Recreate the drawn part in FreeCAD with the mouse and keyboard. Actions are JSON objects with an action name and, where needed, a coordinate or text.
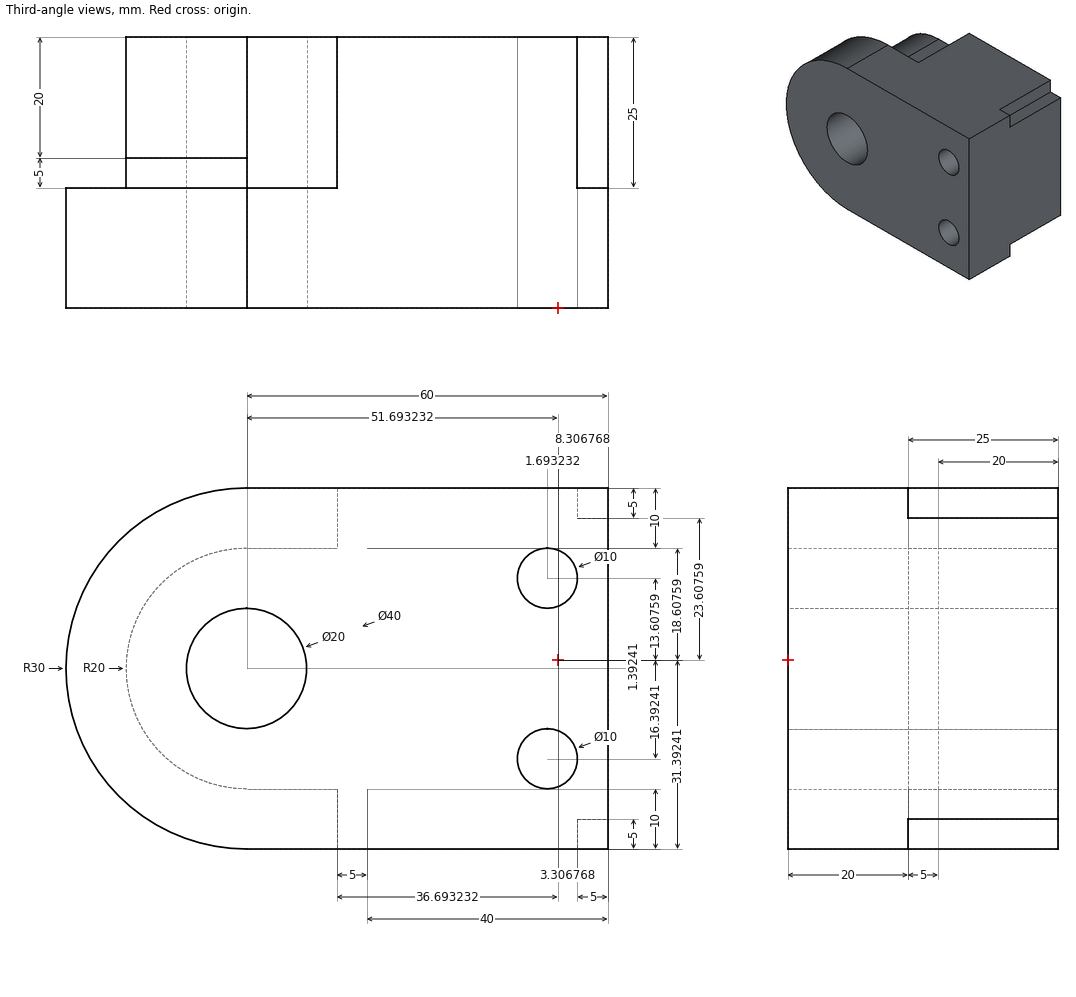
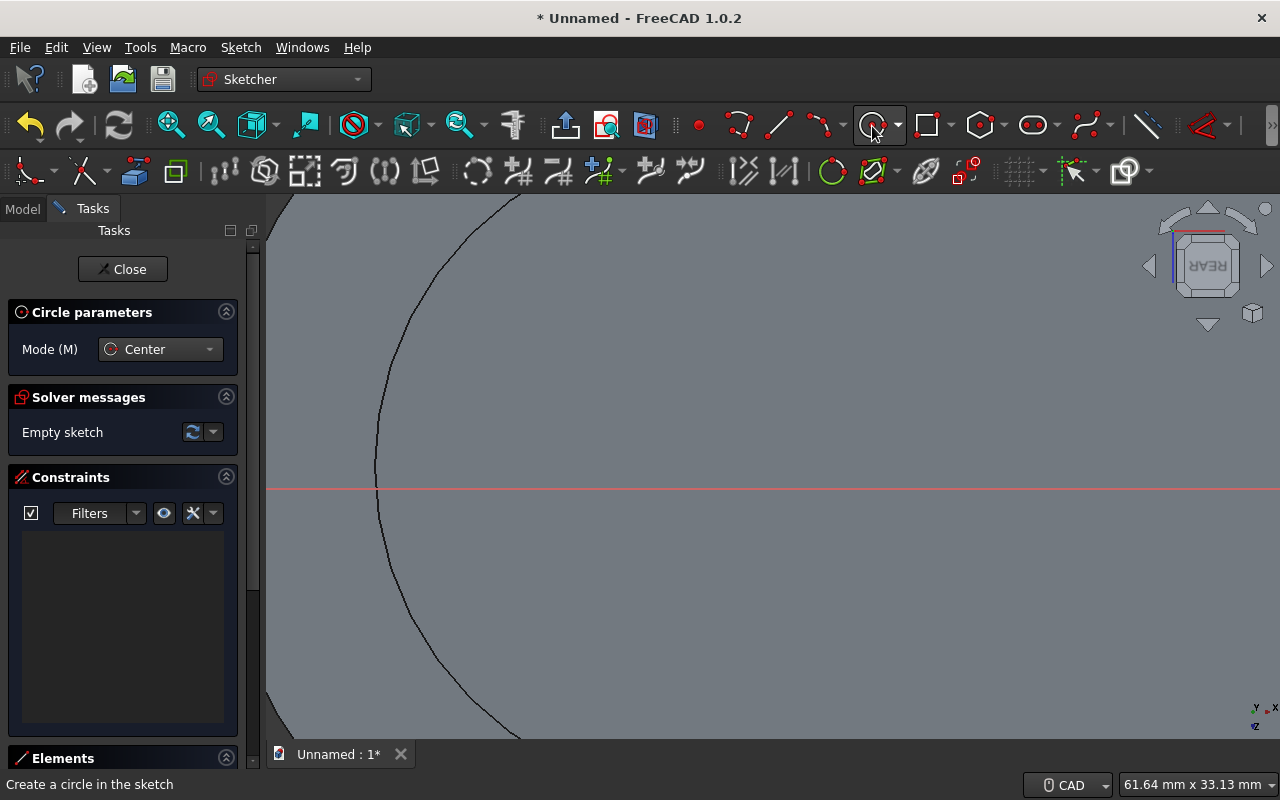
{"action": "left_click", "coordinate": [704, 466]}
{"action": "left_click", "coordinate": [820, 350]}
{"action": "key", "text": "Escape"}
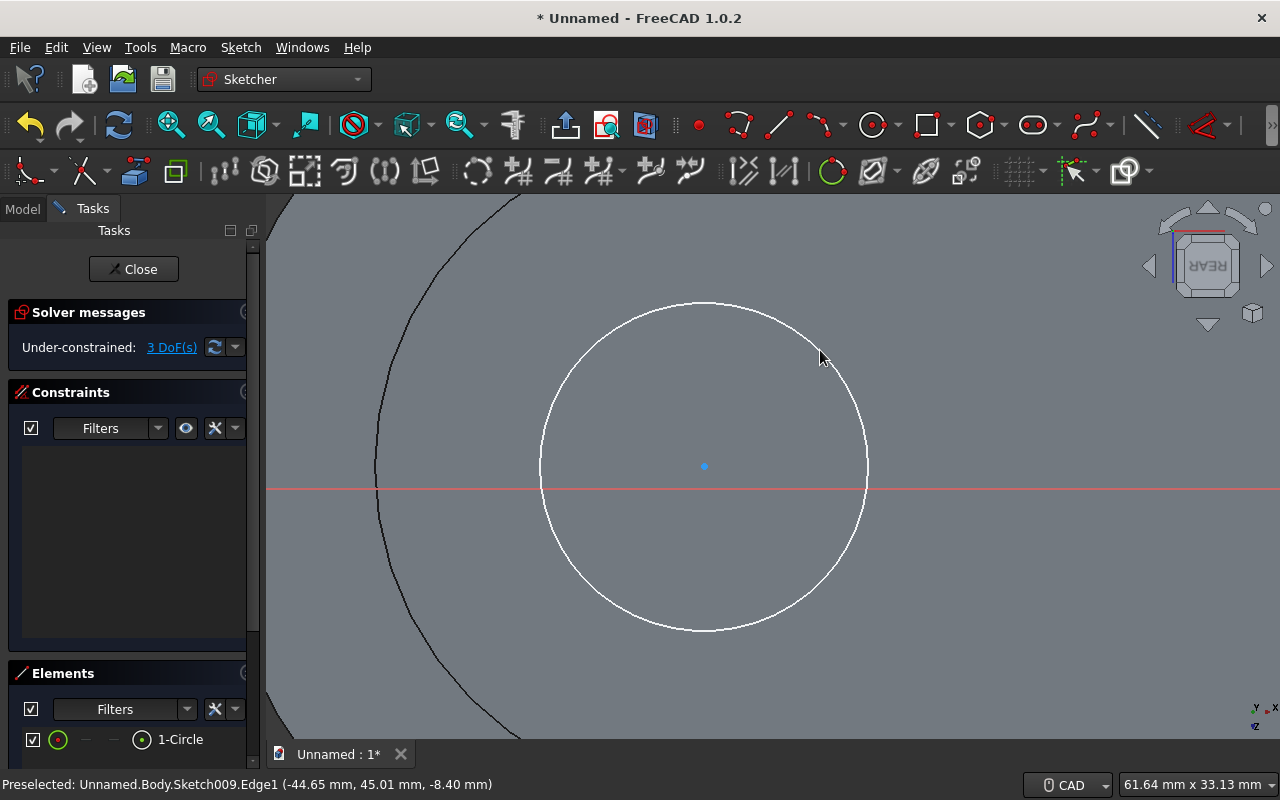
{"action": "left_click", "coordinate": [1202, 126]}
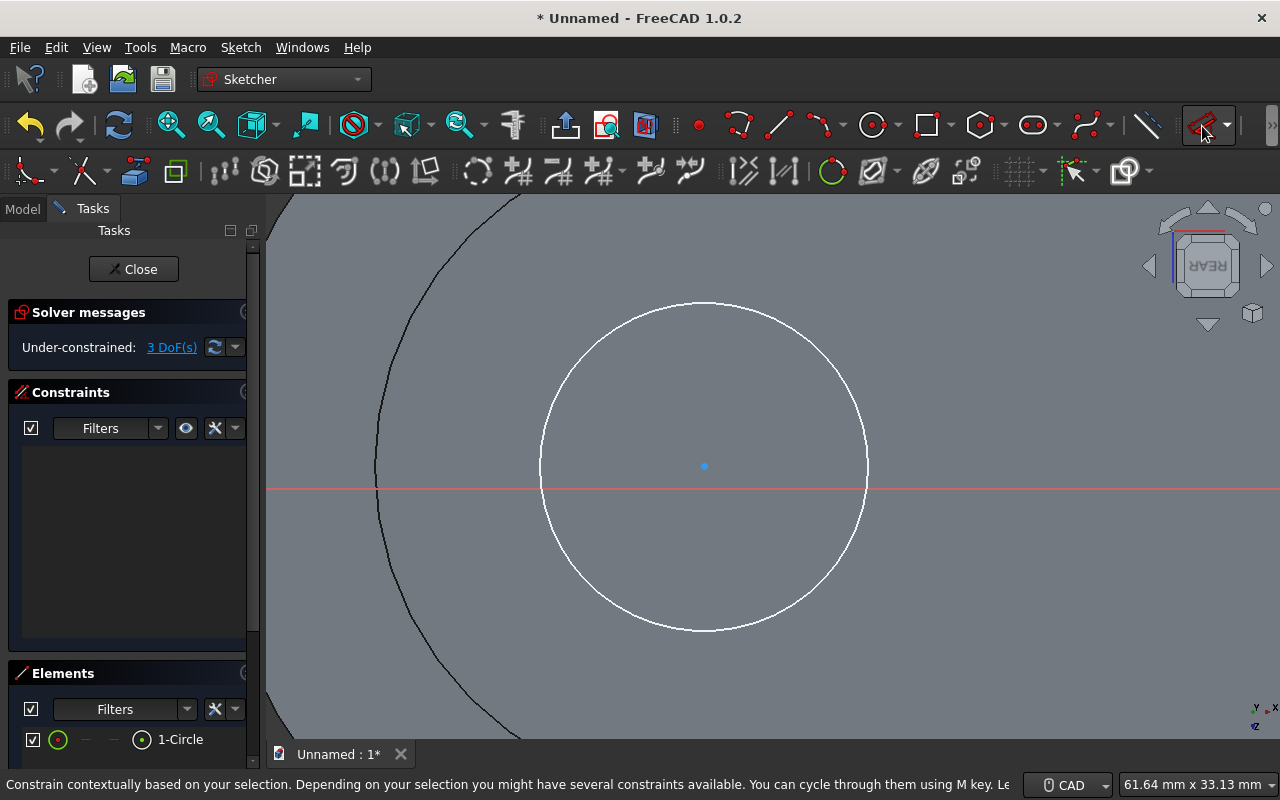
{"action": "left_click", "coordinate": [820, 351]}
{"action": "left_click", "coordinate": [843, 328]}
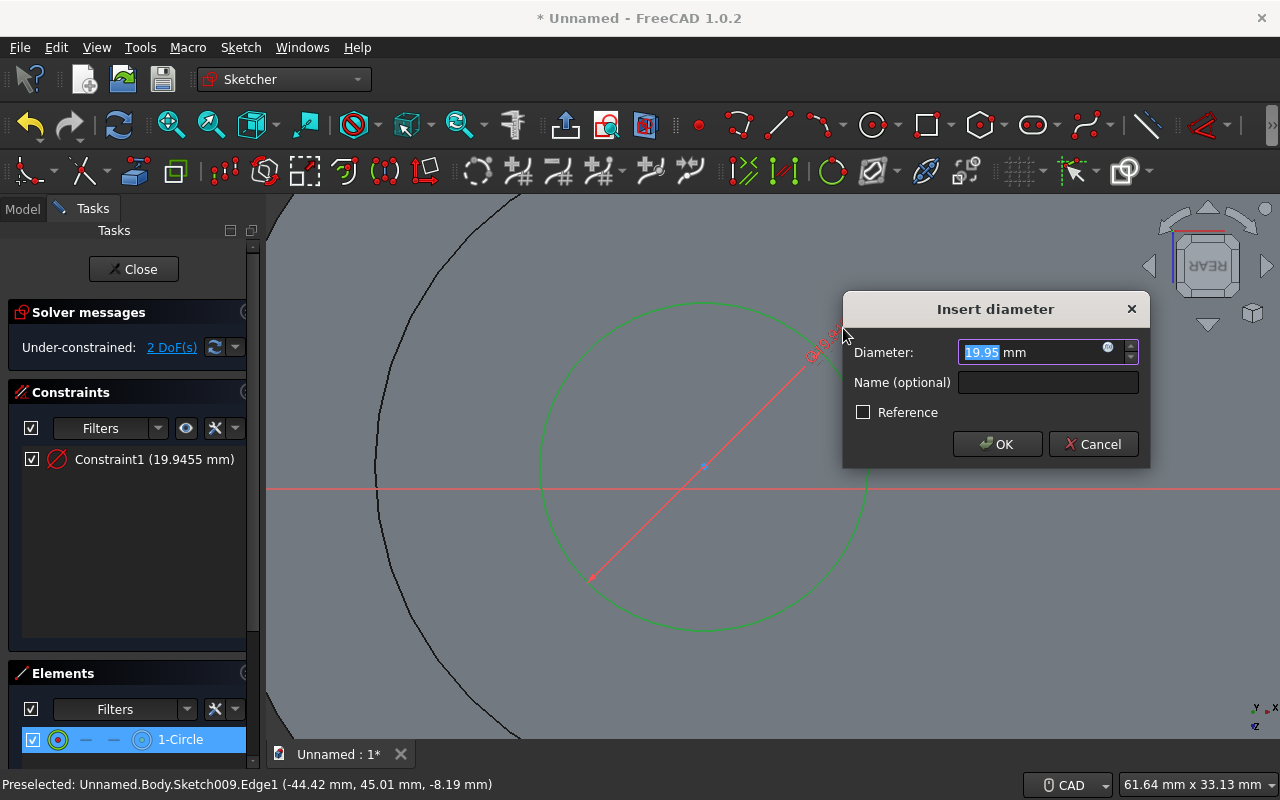
{"action": "type", "text": "20"}
{"action": "key", "text": "Return"}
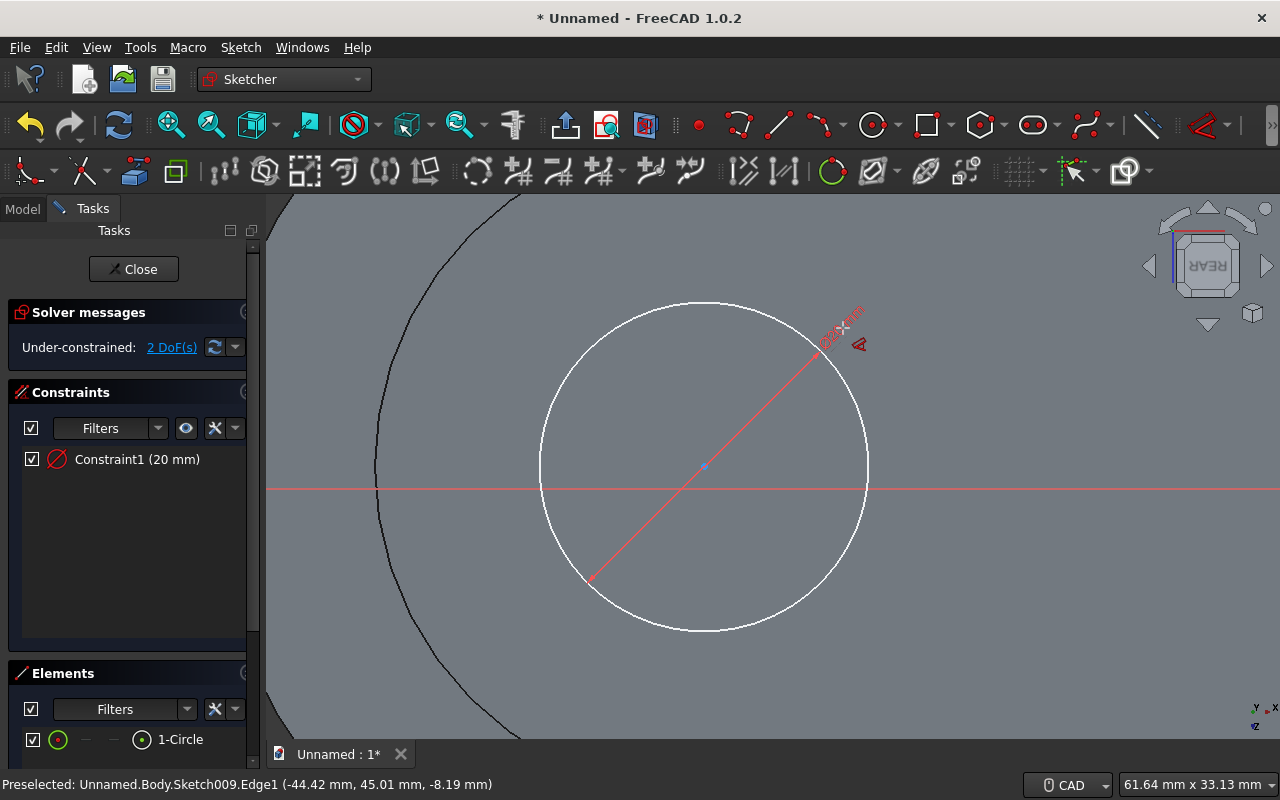
{"action": "scroll", "coordinate": [704, 467], "scroll_direction": "up", "scroll_amount": 3}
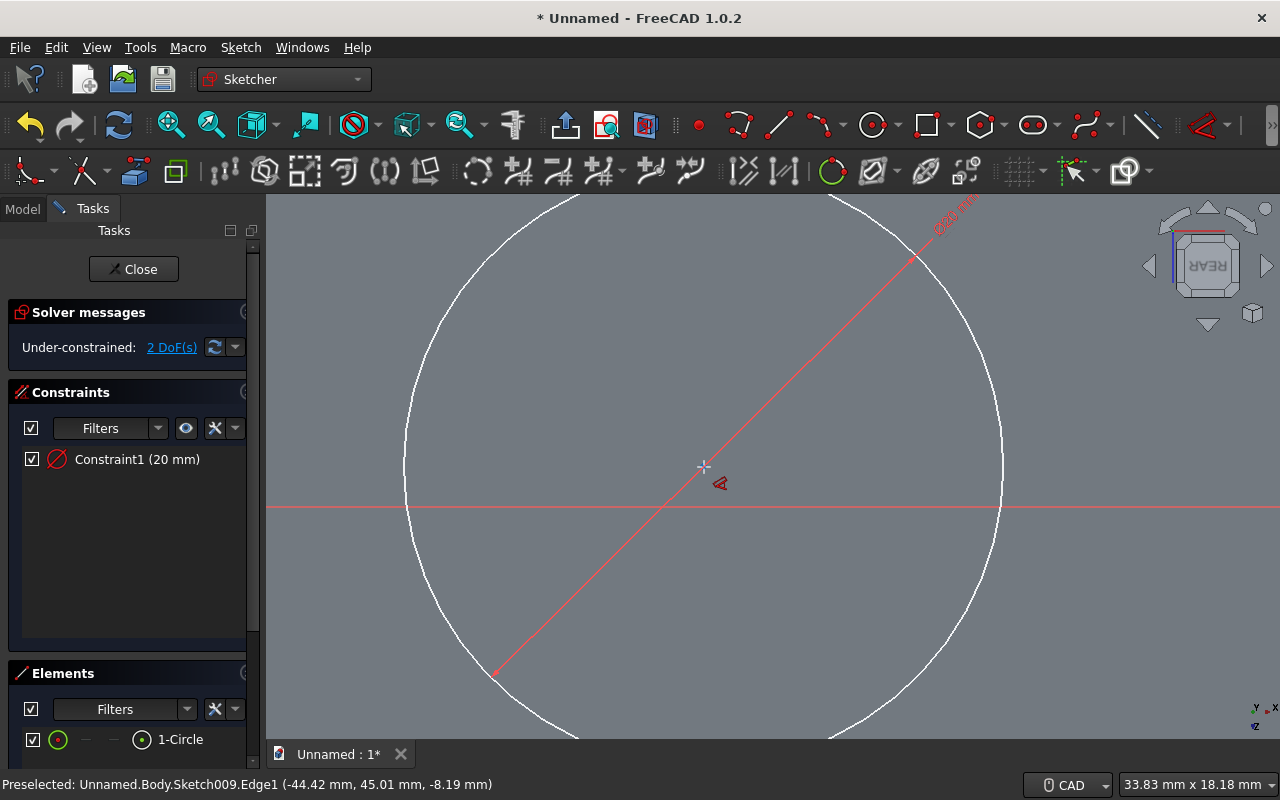
{"action": "left_click", "coordinate": [704, 467]}
{"action": "left_click", "coordinate": [670, 487]}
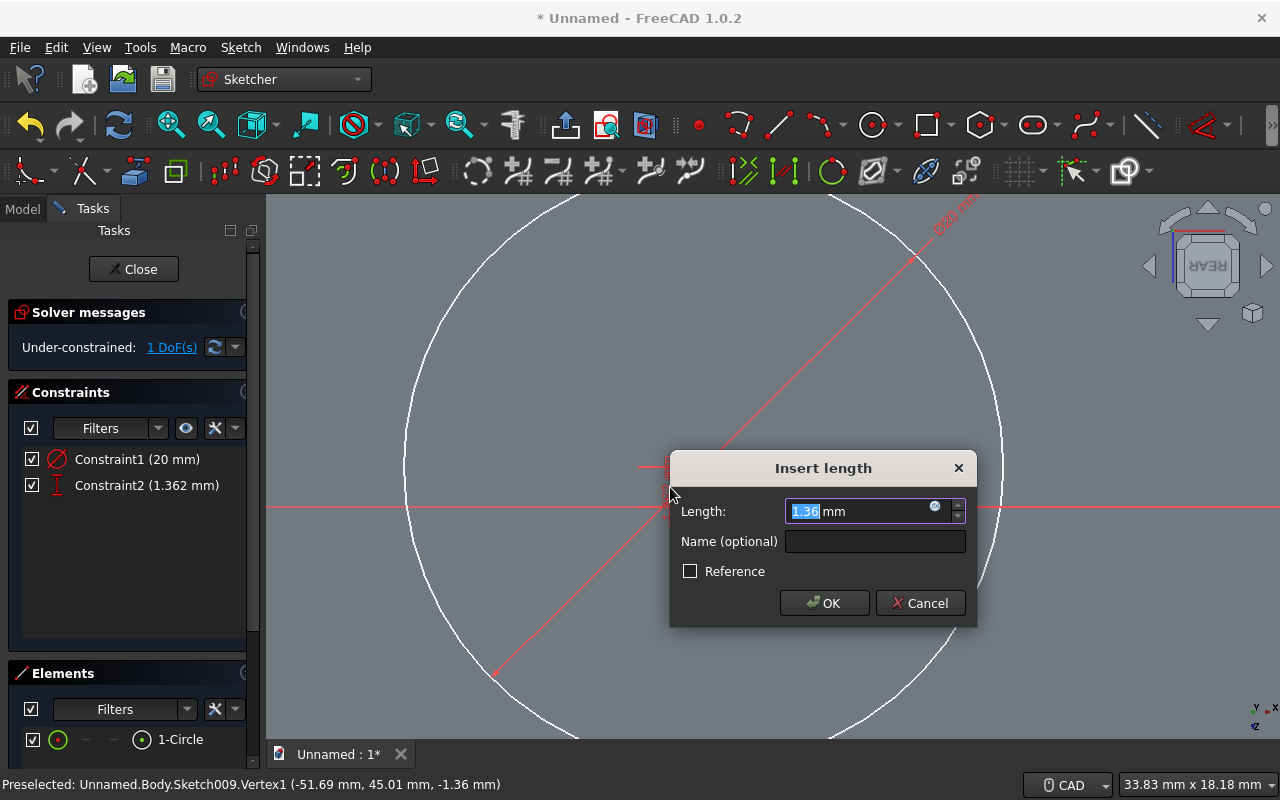
{"action": "type", "text": "1.39241"}
{"action": "key", "text": "Return"}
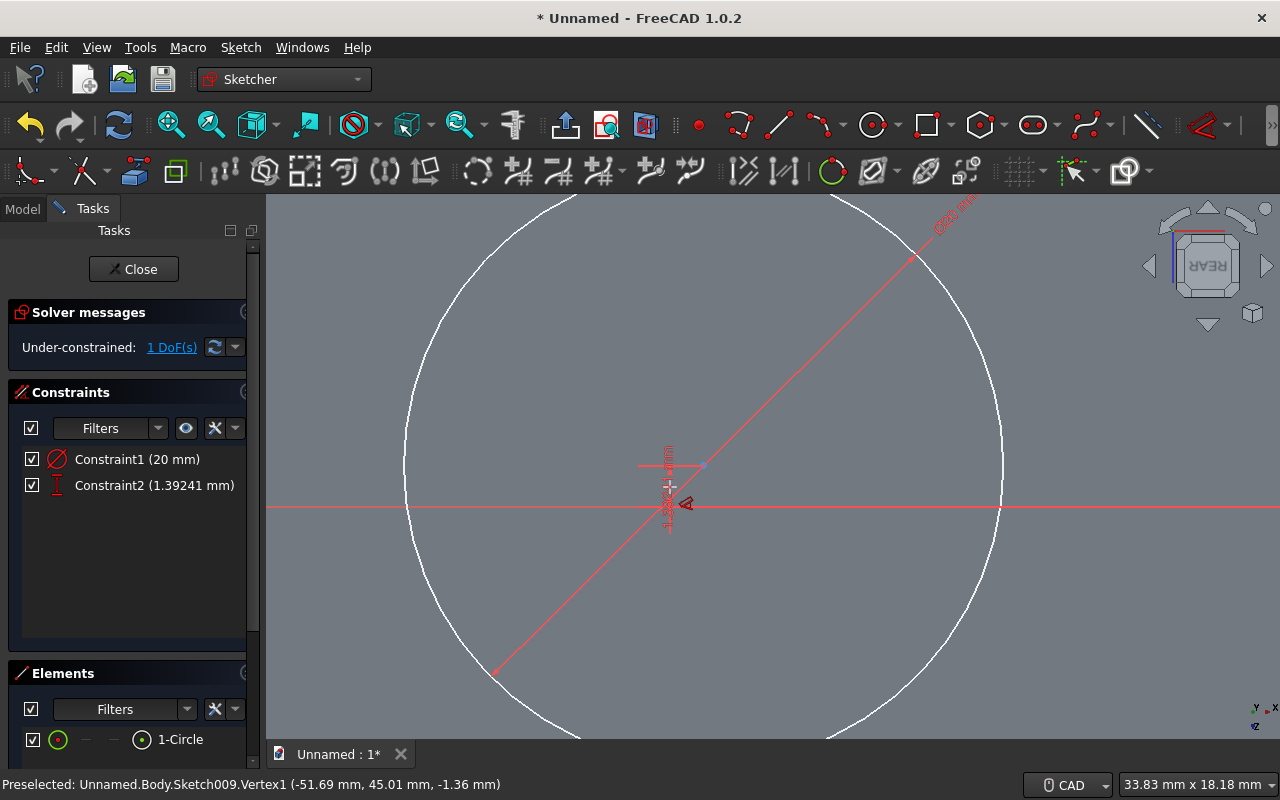
{"action": "left_click", "coordinate": [704, 466]}
{"action": "left_click", "coordinate": [909, 541]}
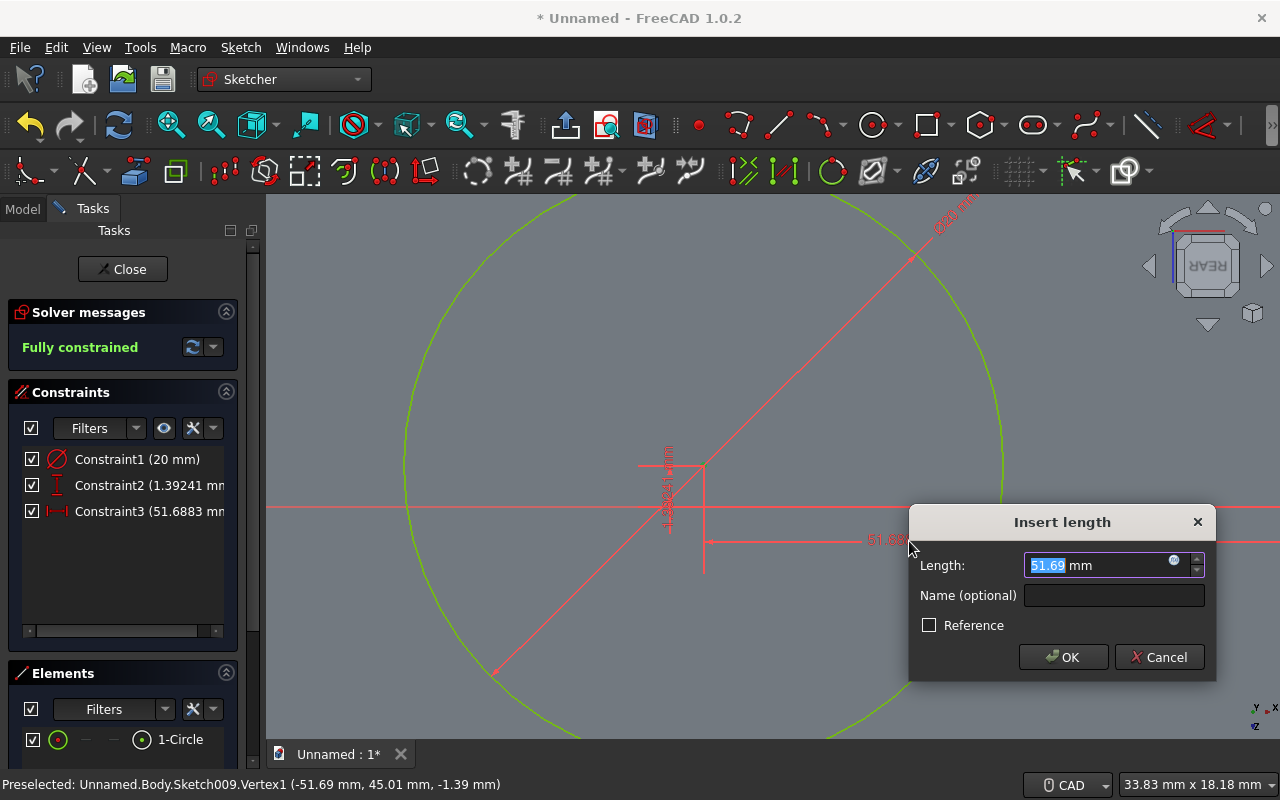
{"action": "type", "text": "51.693232"}
{"action": "key", "text": "Return"}
{"action": "key", "text": "Escape"}